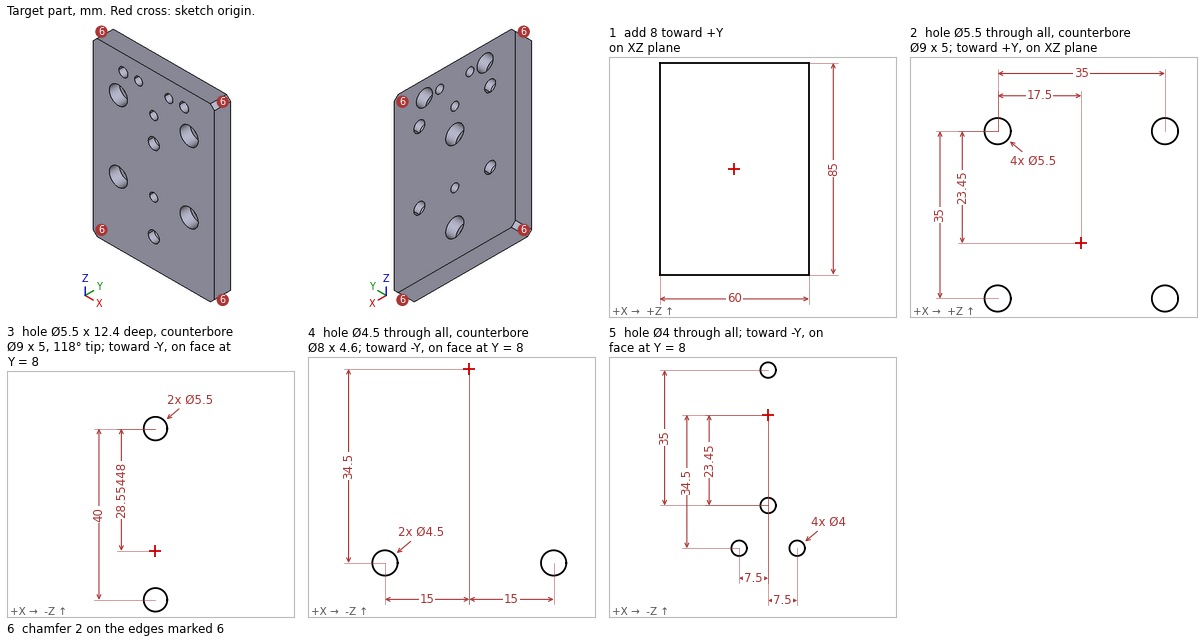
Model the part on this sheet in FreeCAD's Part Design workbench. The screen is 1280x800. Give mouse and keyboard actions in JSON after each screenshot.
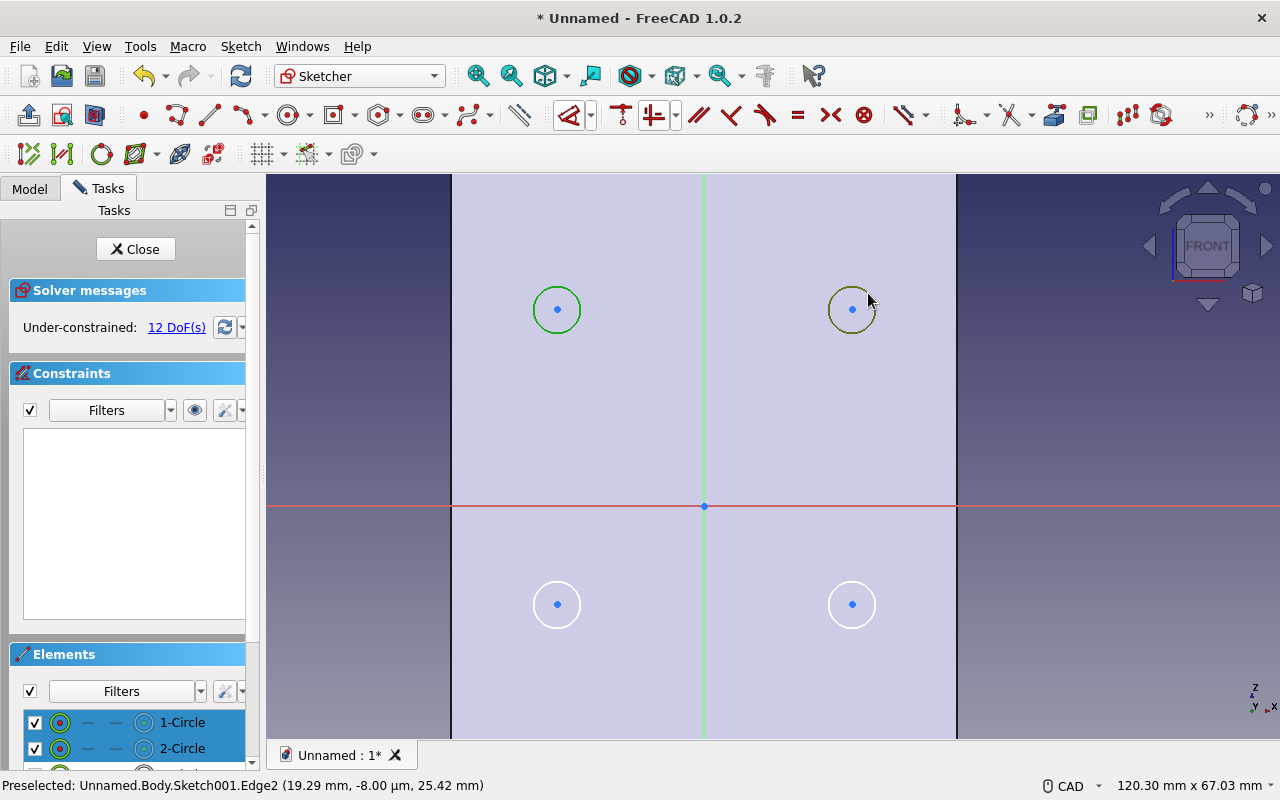
{"action": "left_click", "coordinate": [573, 588]}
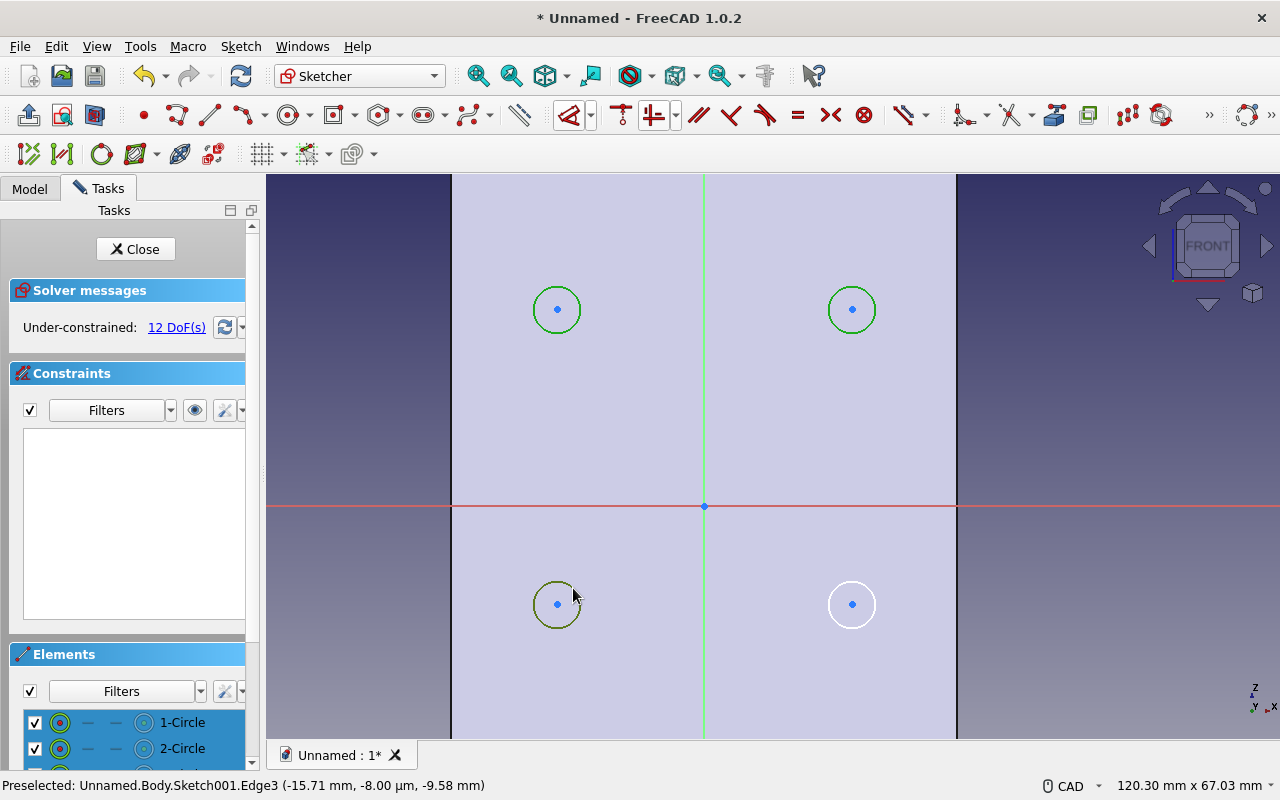
{"action": "left_click", "coordinate": [868, 588]}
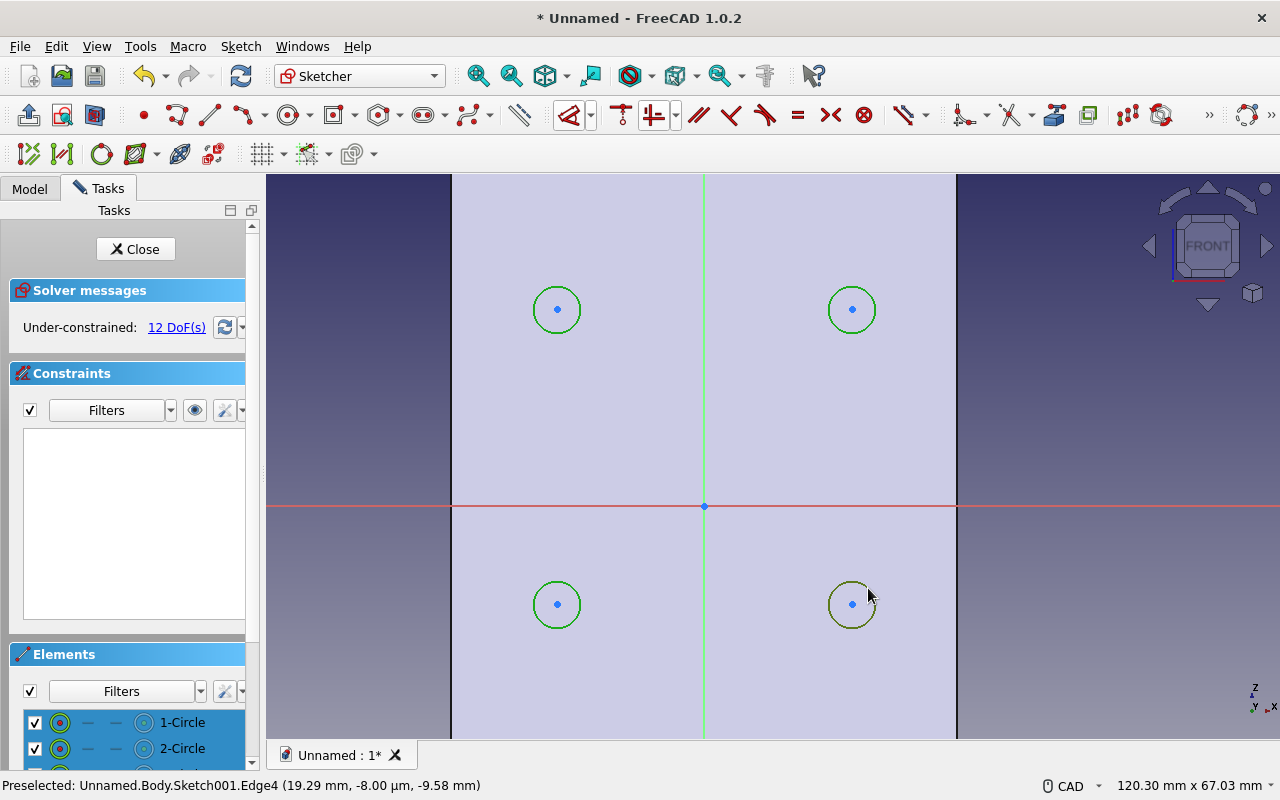
{"action": "left_click", "coordinate": [798, 116]}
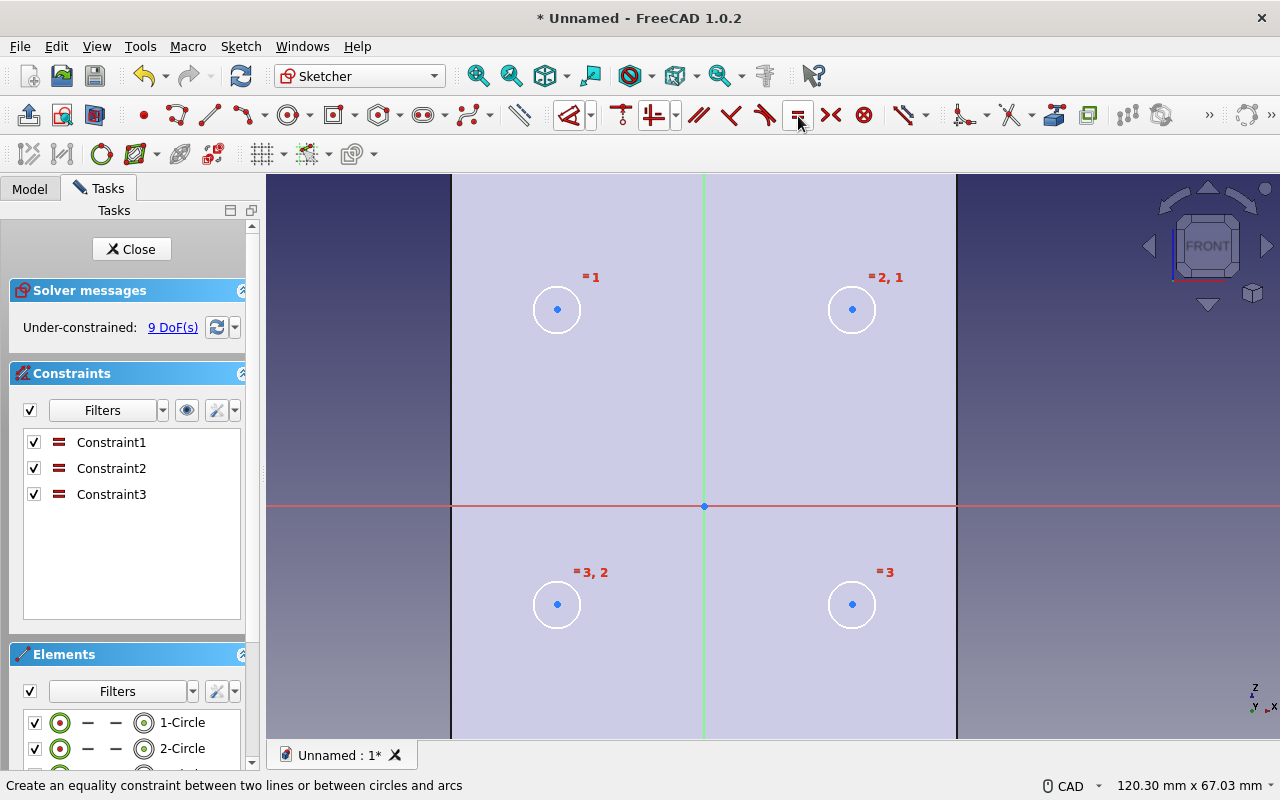
{"action": "left_click", "coordinate": [557, 310]}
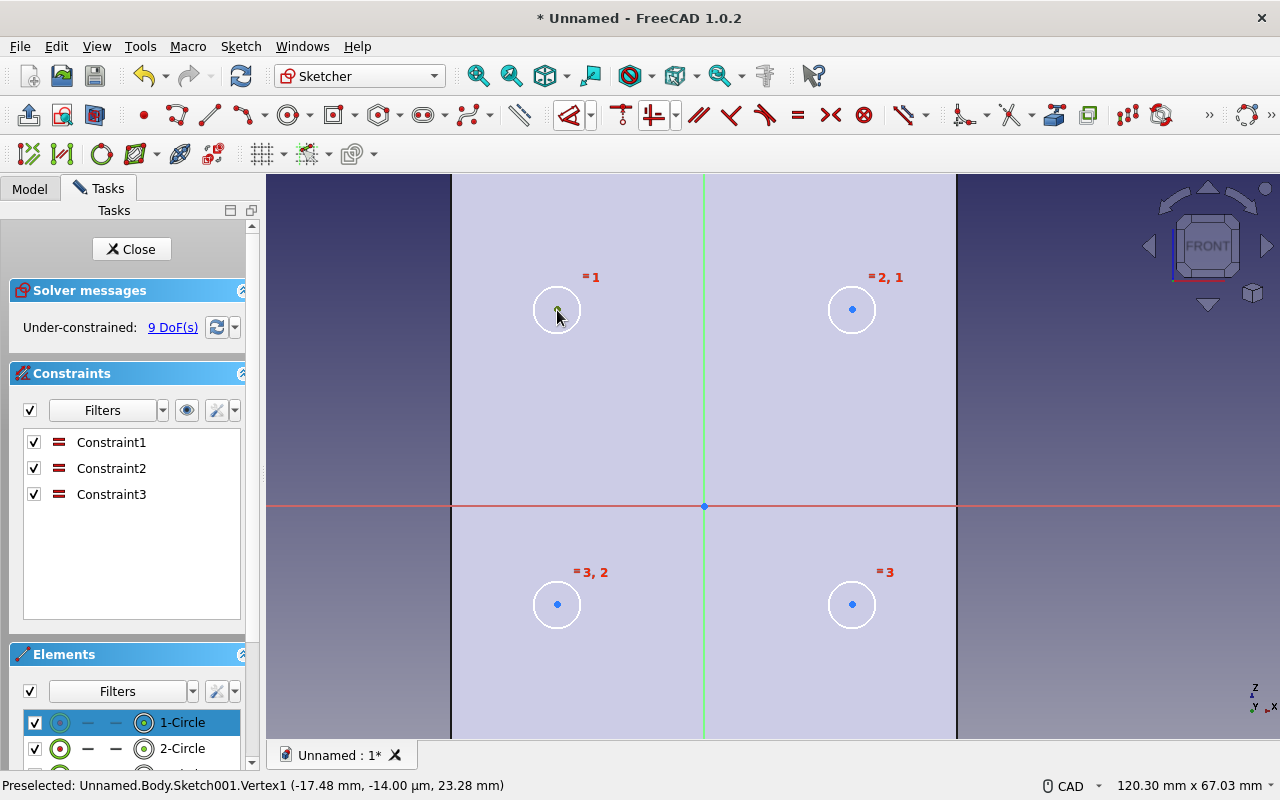
{"action": "left_click", "coordinate": [852, 310]}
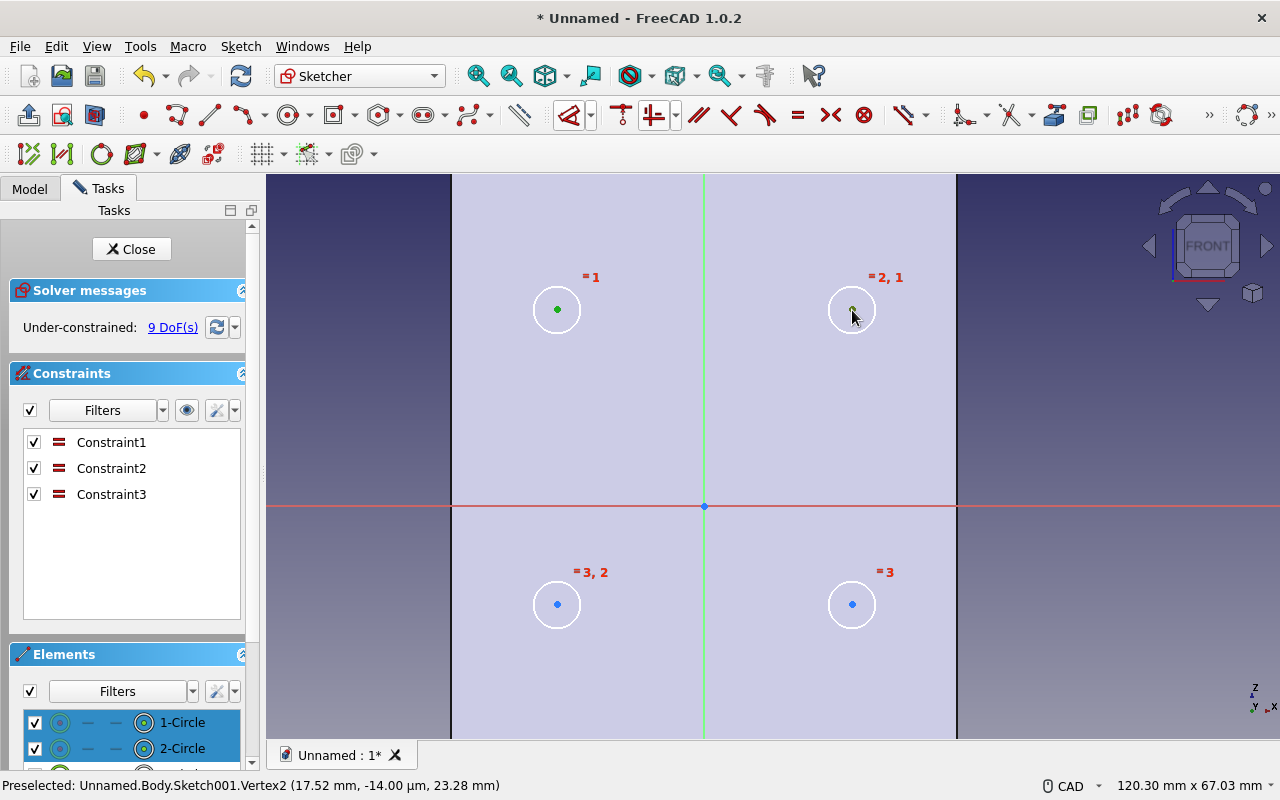
{"action": "left_click", "coordinate": [676, 116]}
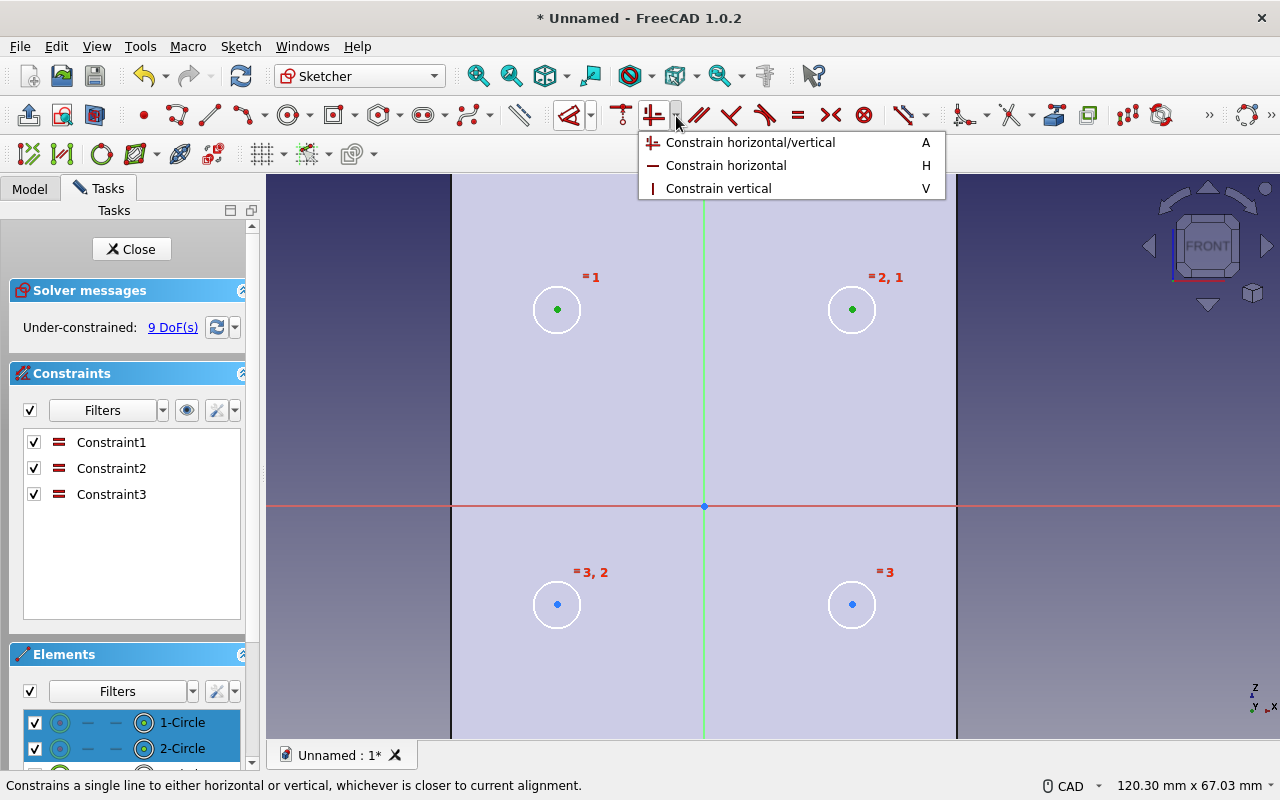
{"action": "left_click", "coordinate": [792, 166]}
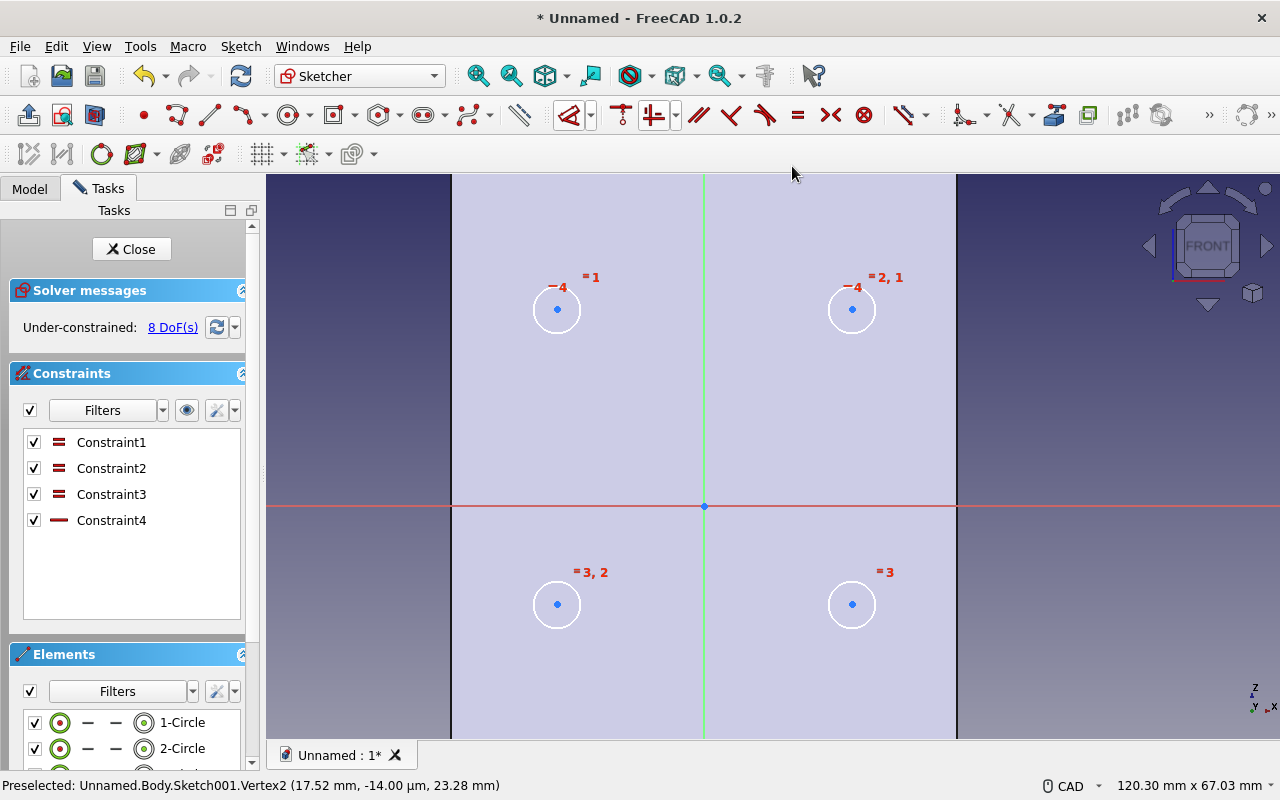
{"action": "left_click", "coordinate": [557, 310]}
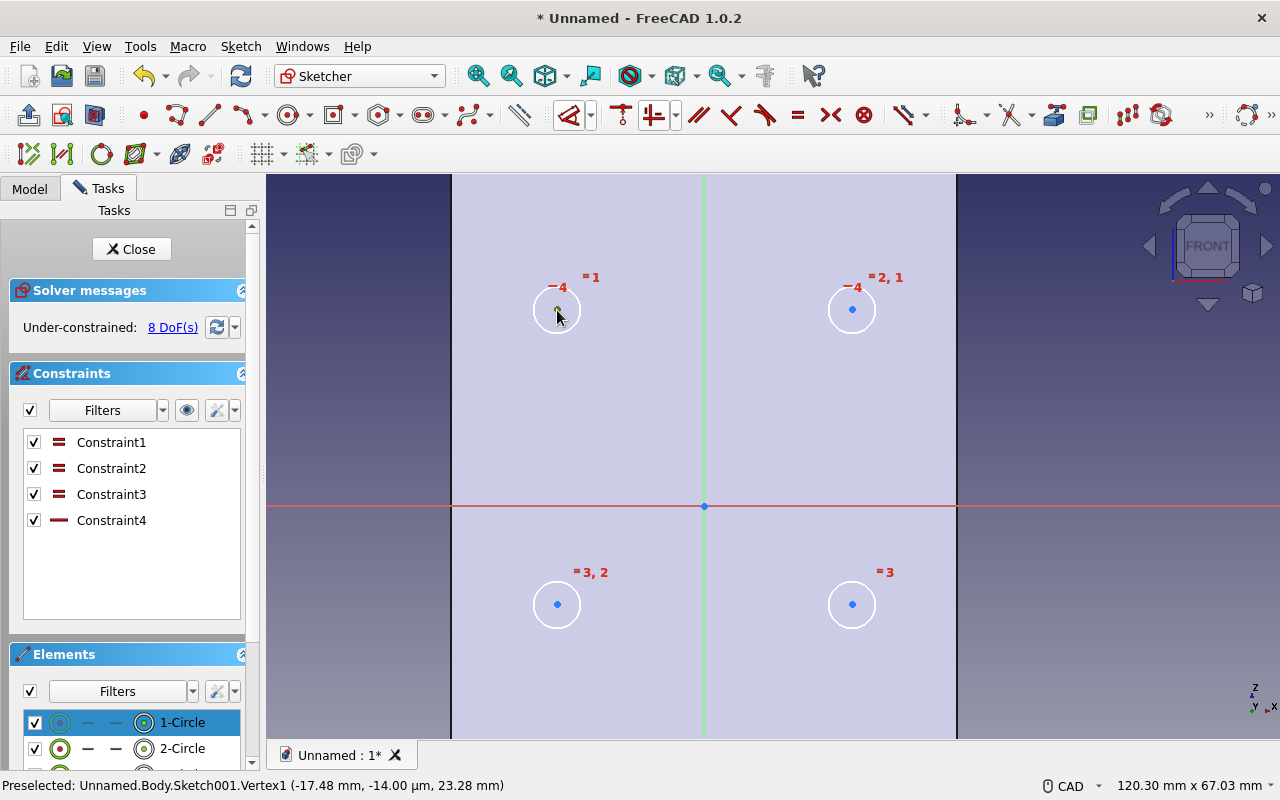
{"action": "left_click", "coordinate": [557, 605]}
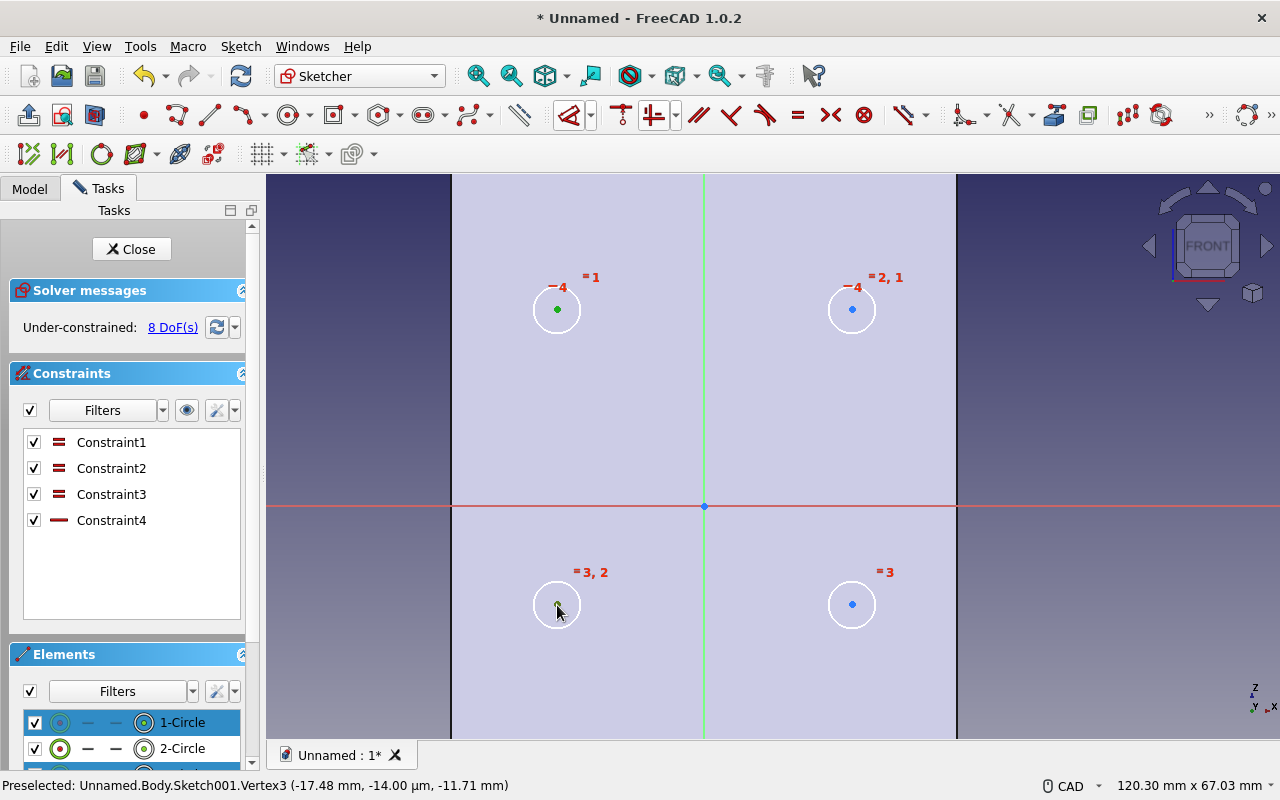
{"action": "left_click", "coordinate": [676, 116]}